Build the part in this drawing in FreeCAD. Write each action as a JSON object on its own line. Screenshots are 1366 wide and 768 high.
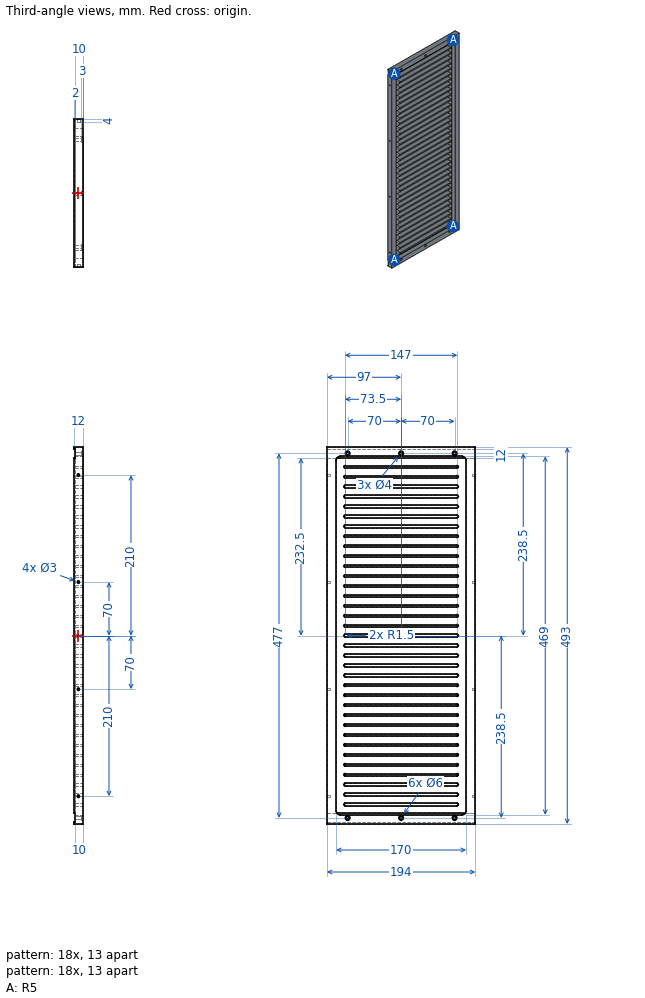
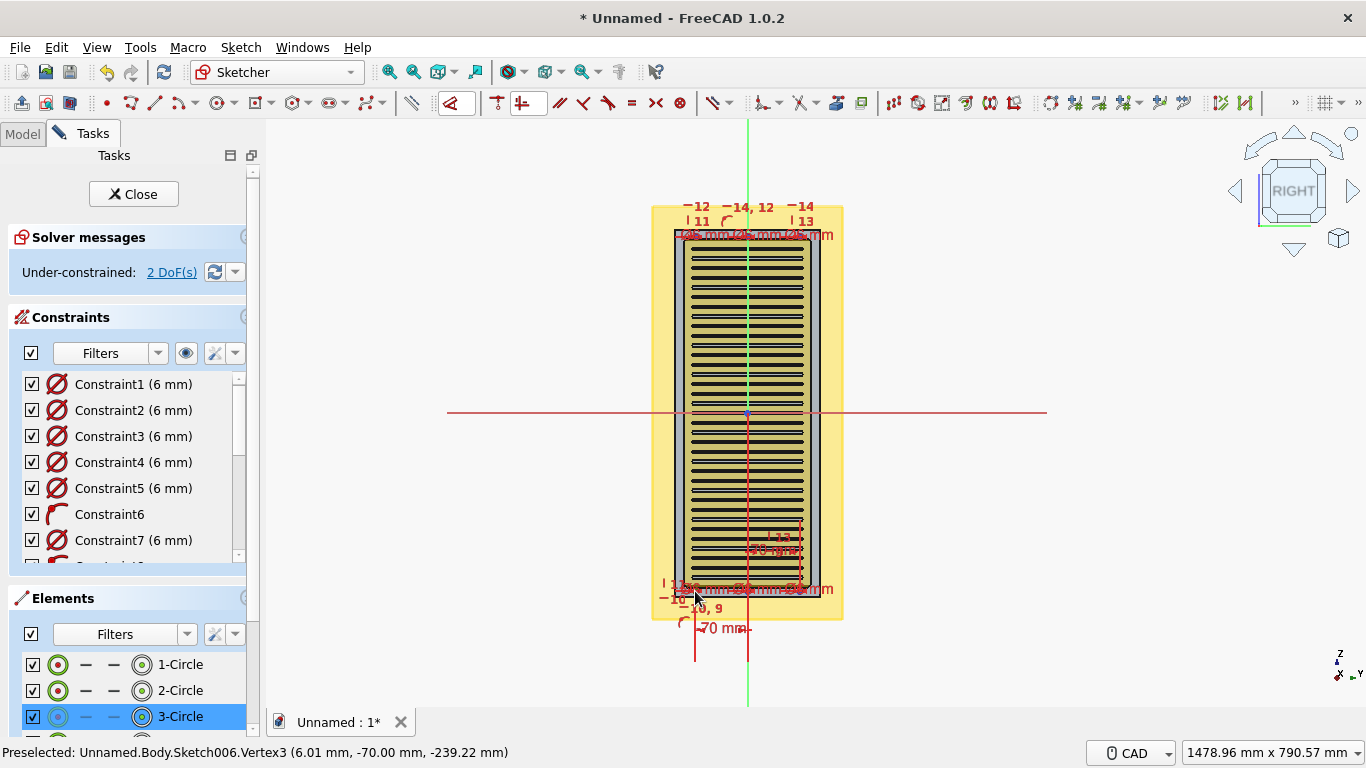
{"action": "left_click", "coordinate": [695, 237]}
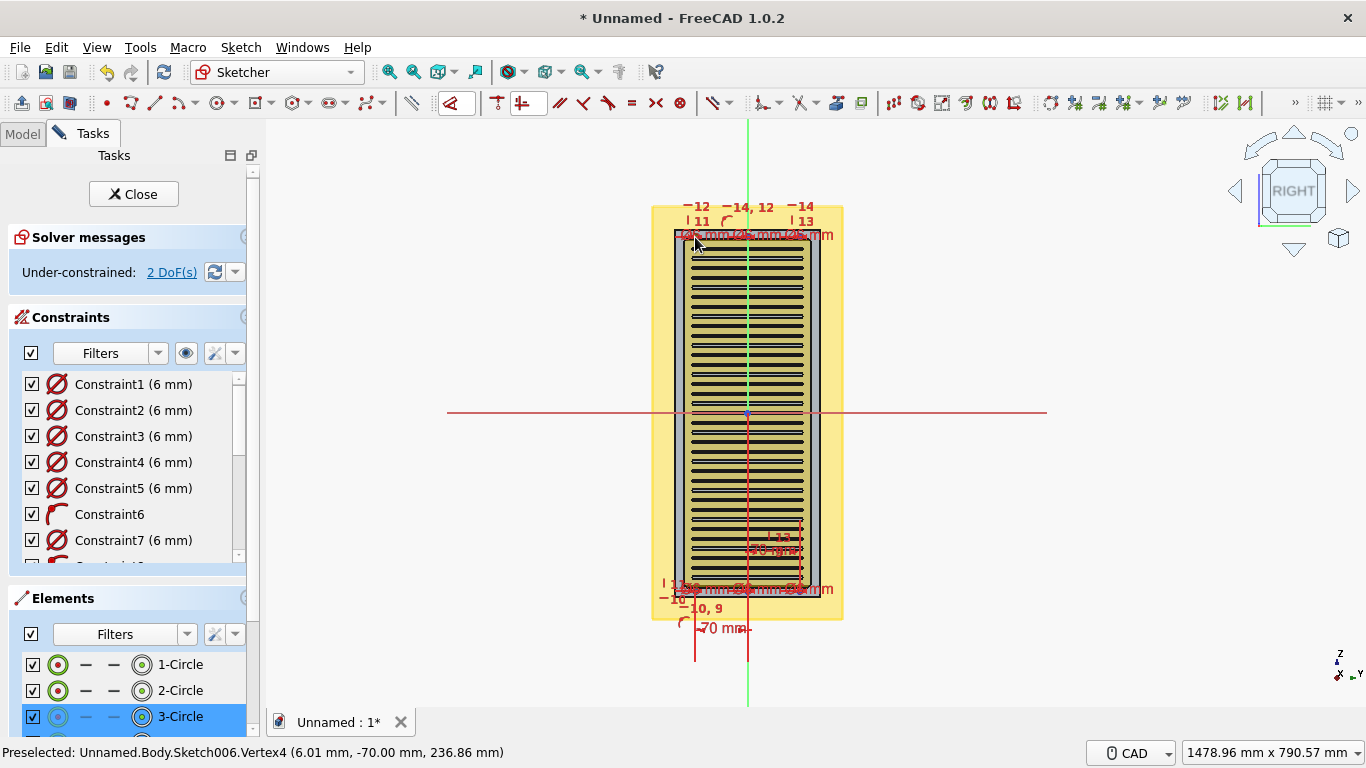
{"action": "key", "text": "i"}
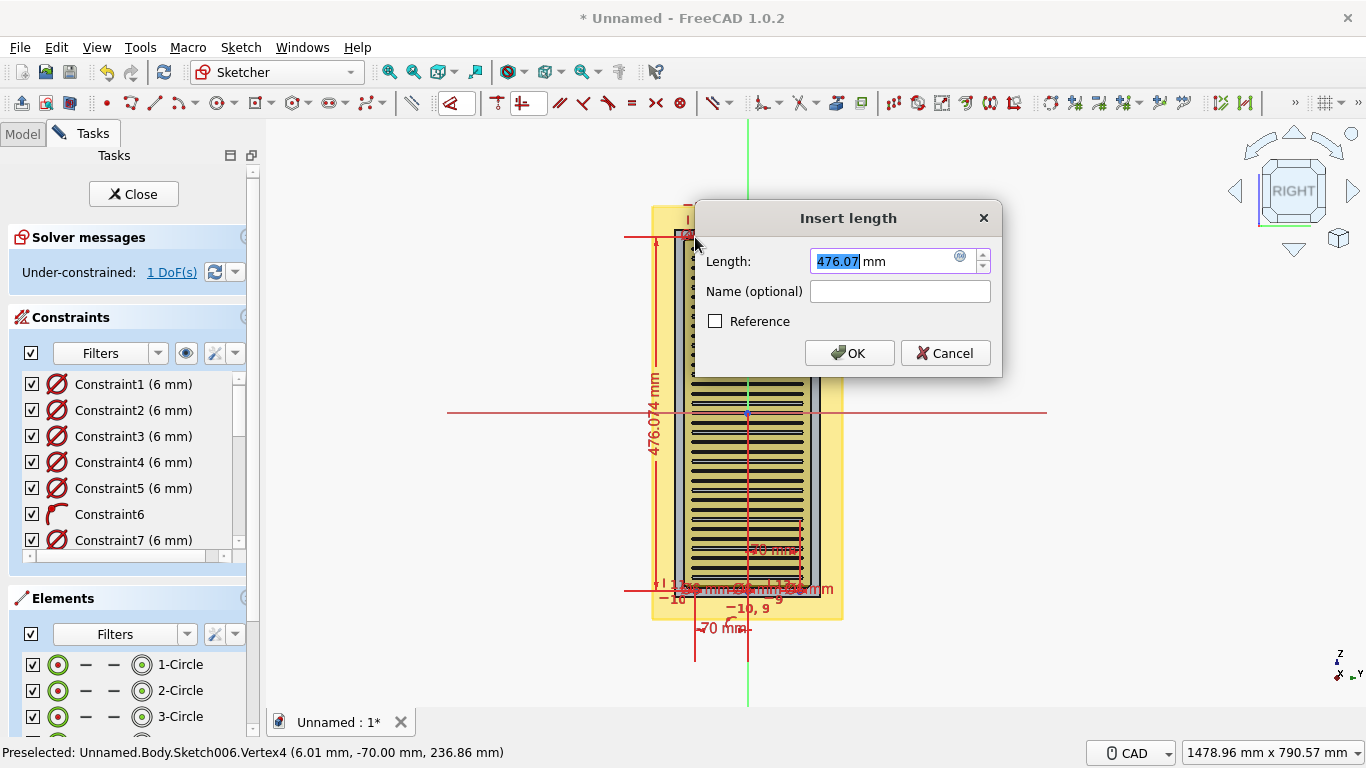
{"action": "type", "text": "477"}
{"action": "key", "text": "Return"}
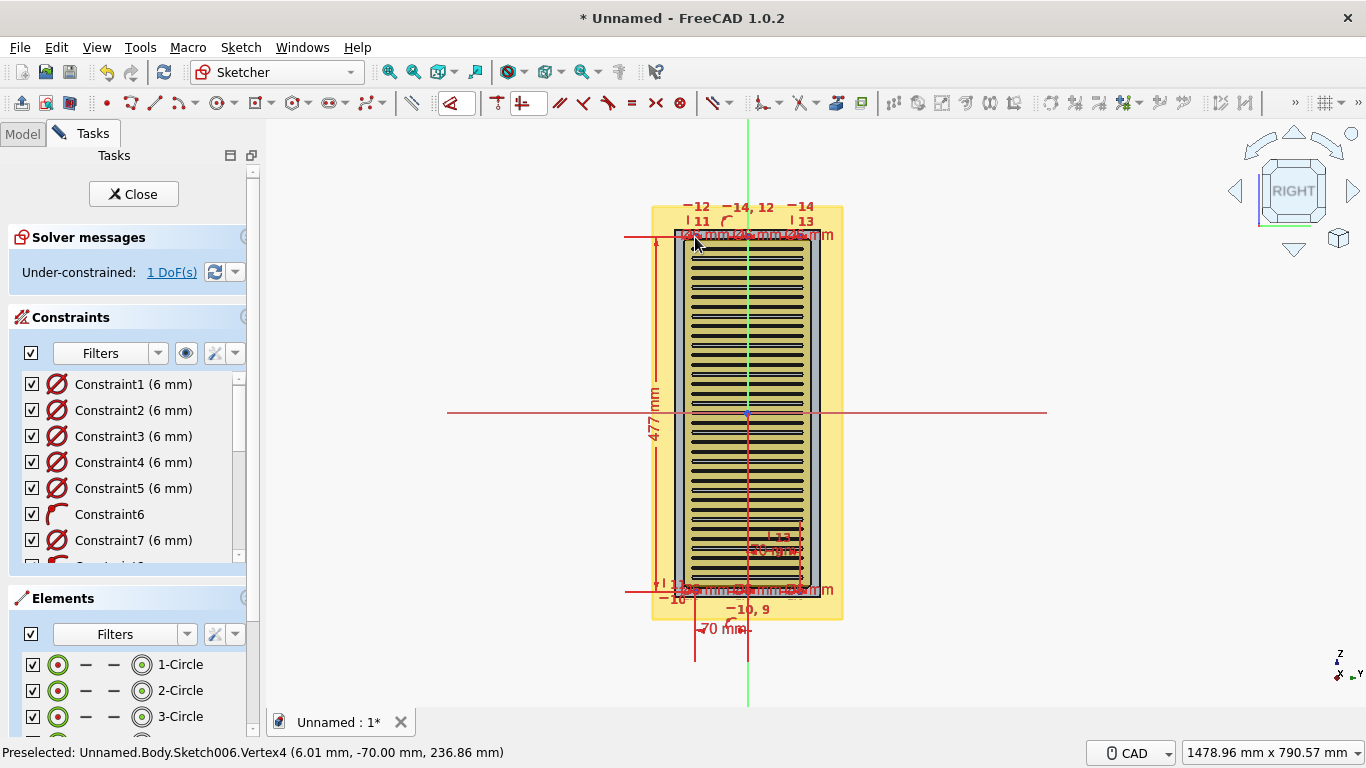
{"action": "left_click", "coordinate": [748, 592]}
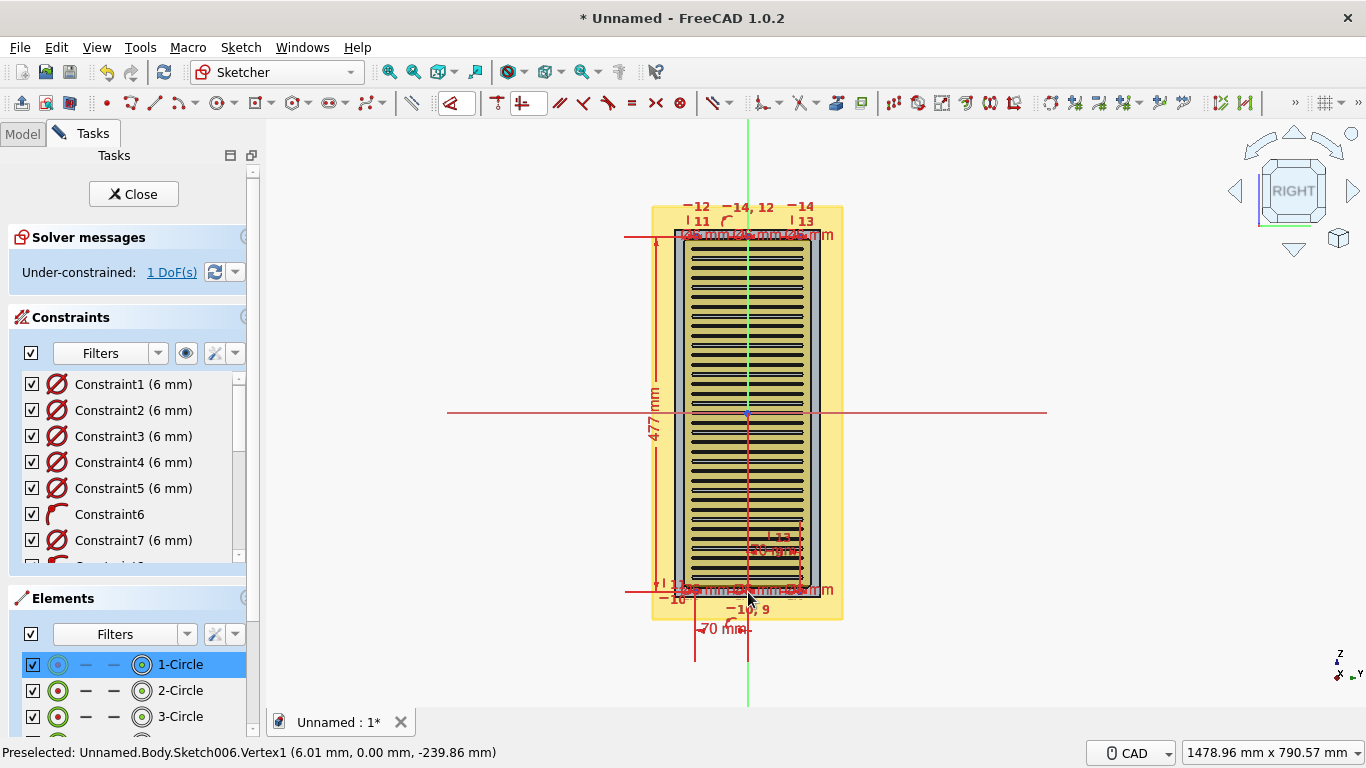
{"action": "left_click", "coordinate": [470, 104]}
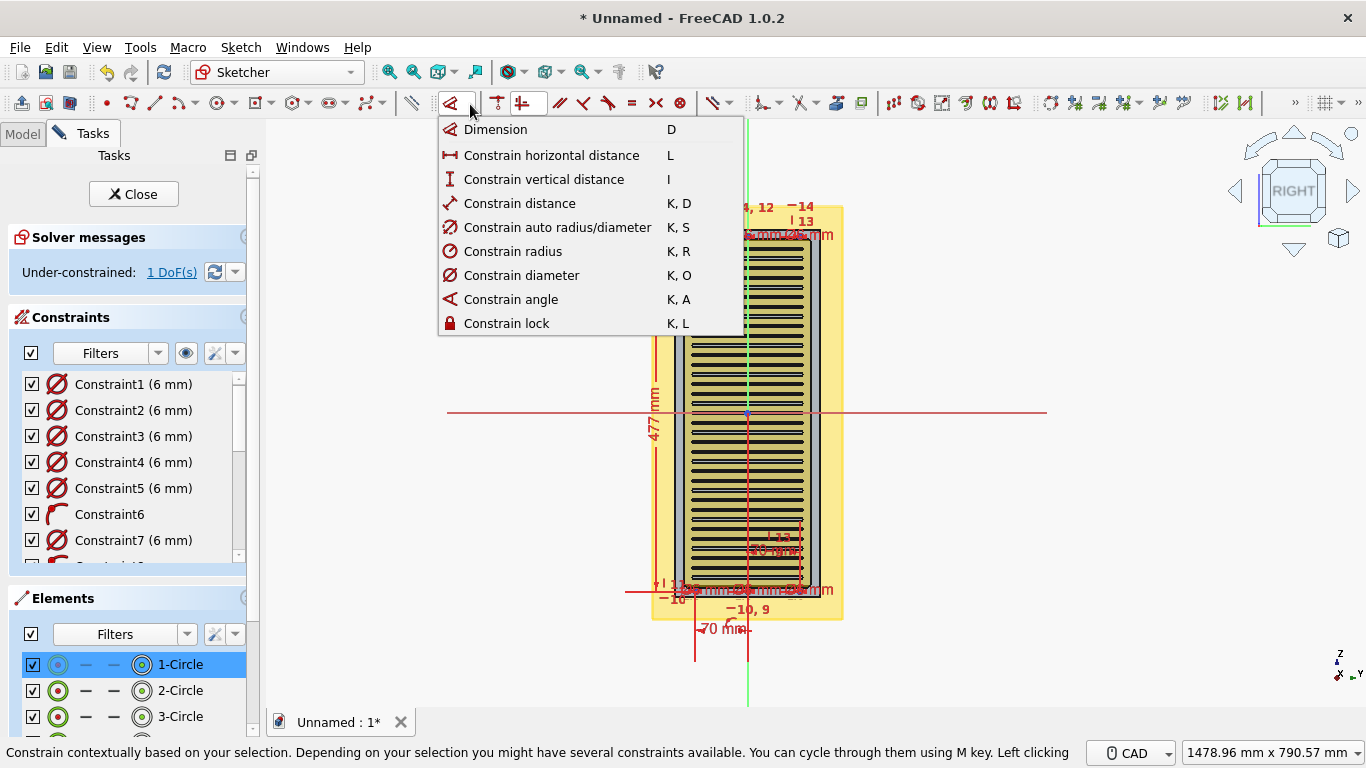
{"action": "left_click", "coordinate": [591, 179]}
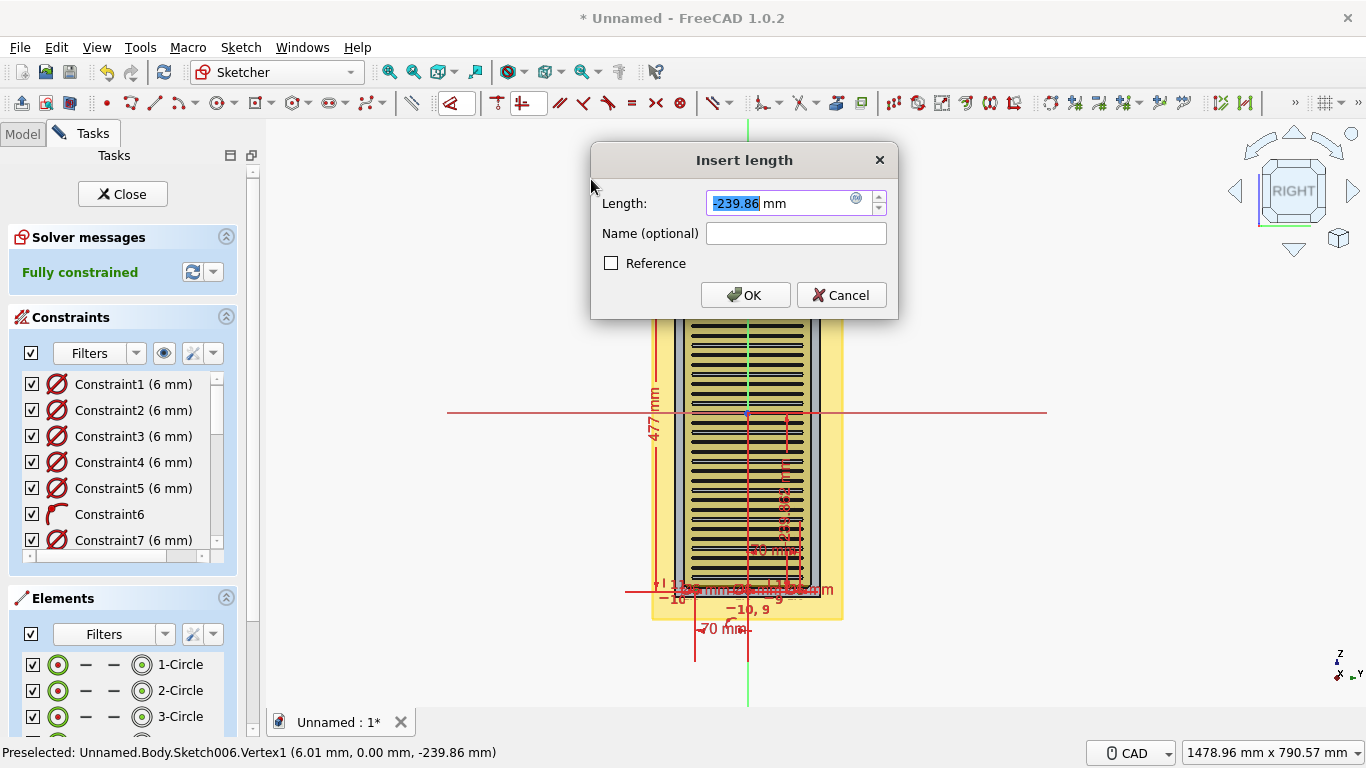
{"action": "type", "text": "-238.5"}
{"action": "key", "text": "Return"}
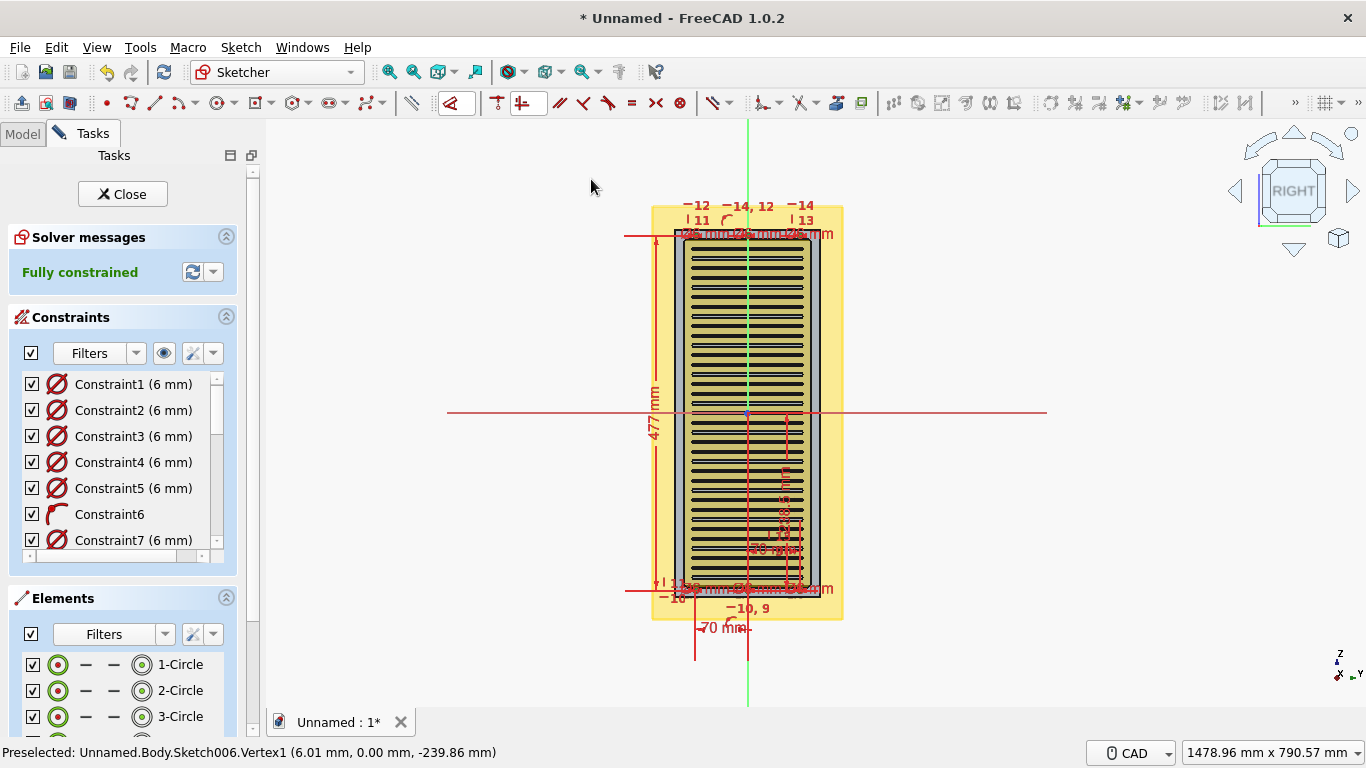
{"action": "left_click", "coordinate": [123, 194]}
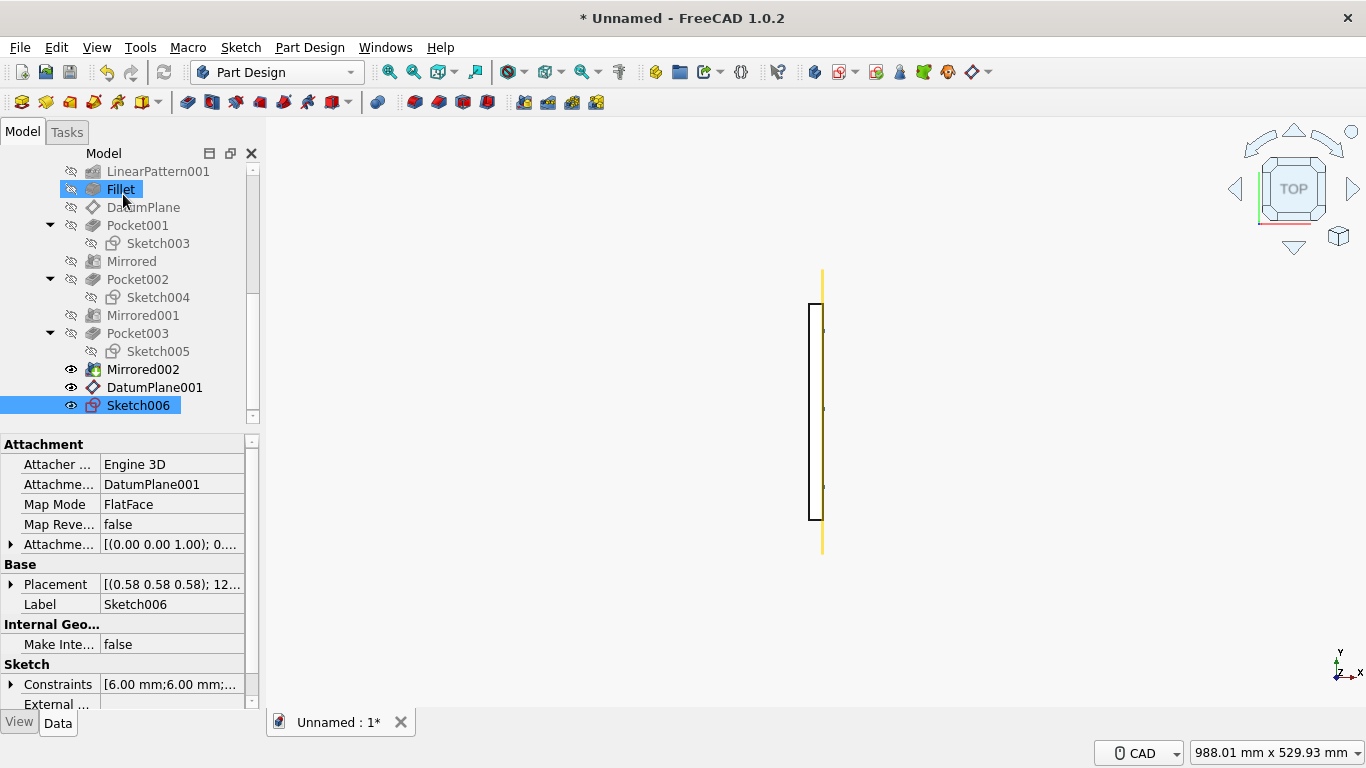
{"action": "left_click", "coordinate": [188, 102]}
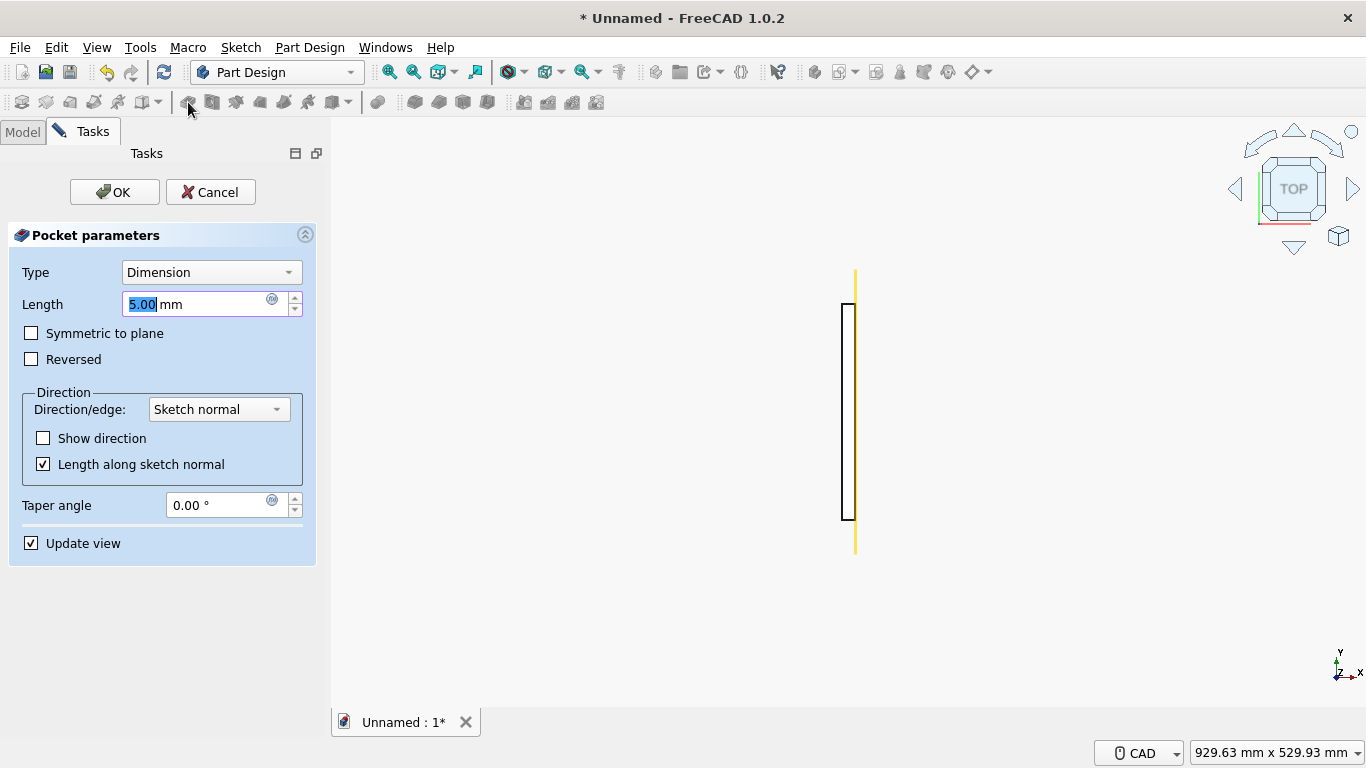
{"action": "type", "text": "3"}
{"action": "key", "text": "Tab"}